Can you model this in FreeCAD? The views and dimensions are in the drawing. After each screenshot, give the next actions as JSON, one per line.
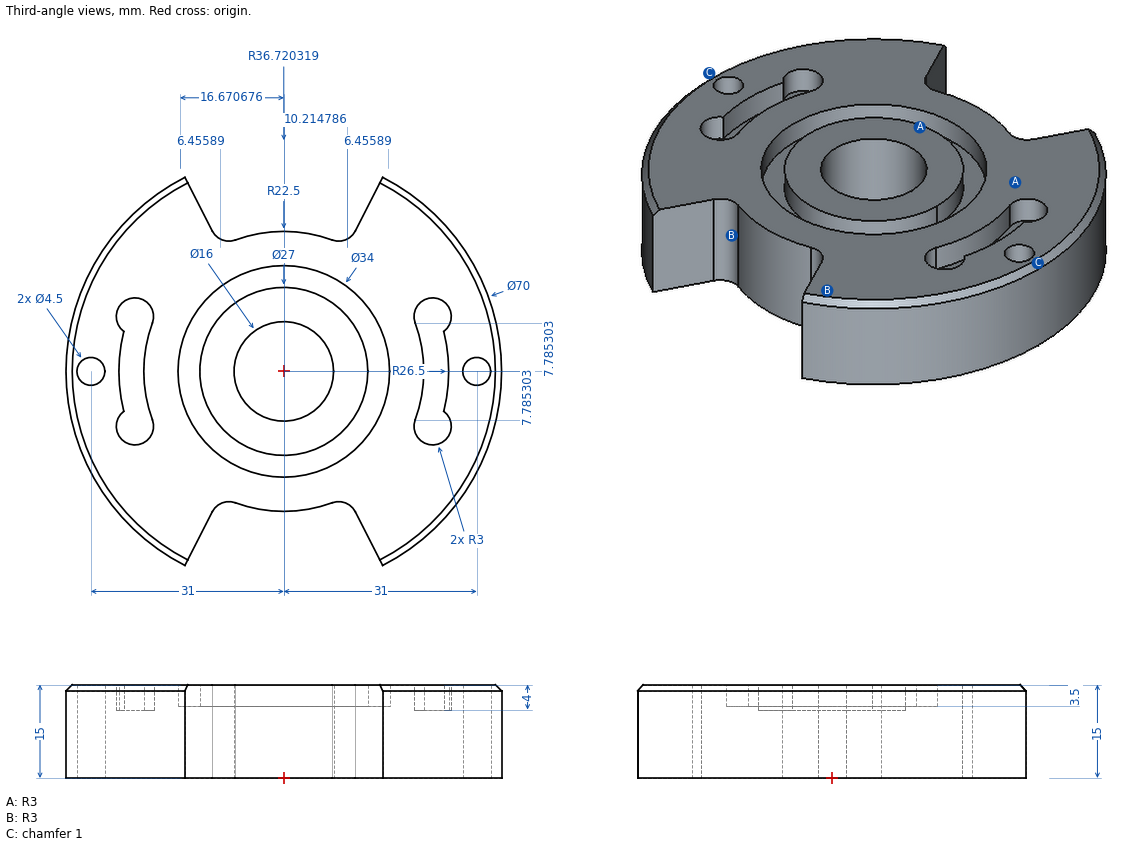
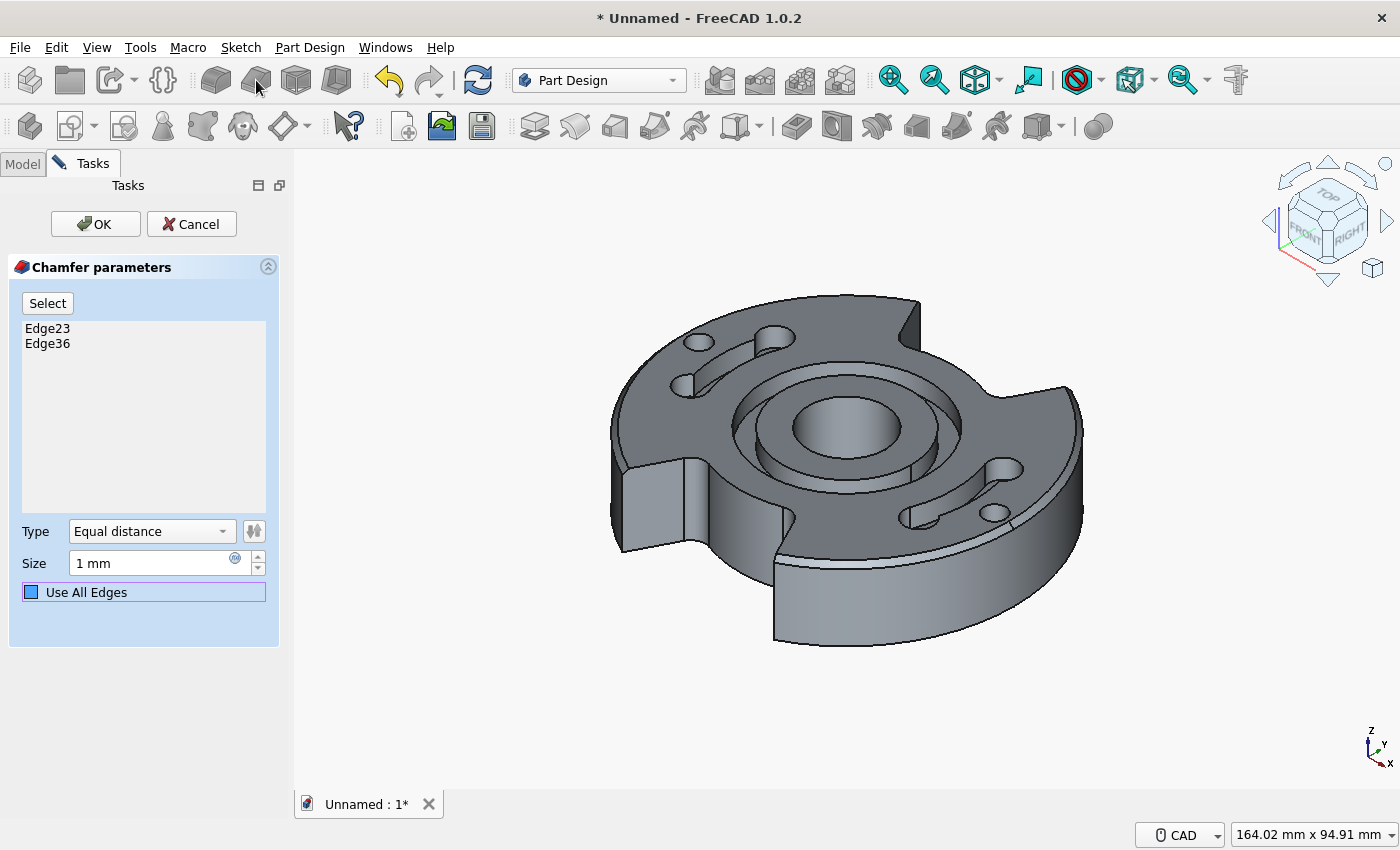
{"action": "left_click", "coordinate": [96, 224]}